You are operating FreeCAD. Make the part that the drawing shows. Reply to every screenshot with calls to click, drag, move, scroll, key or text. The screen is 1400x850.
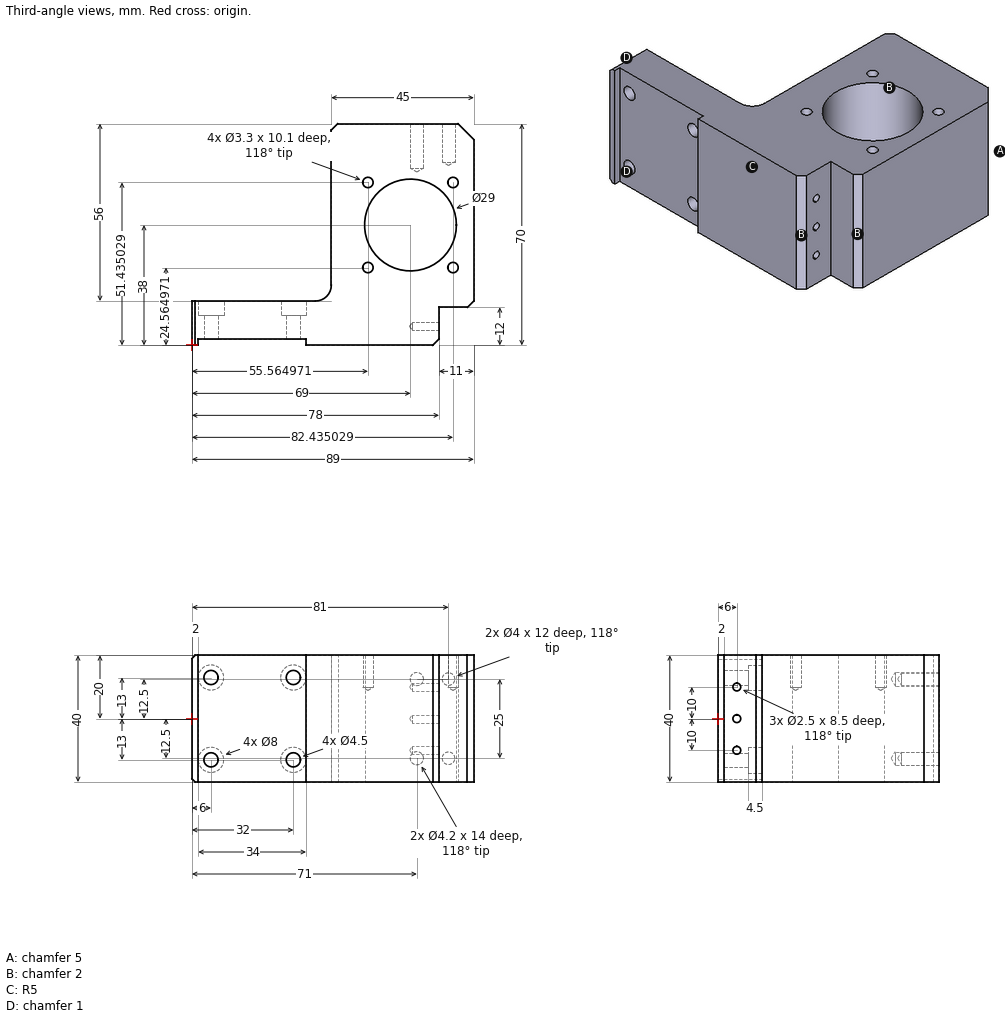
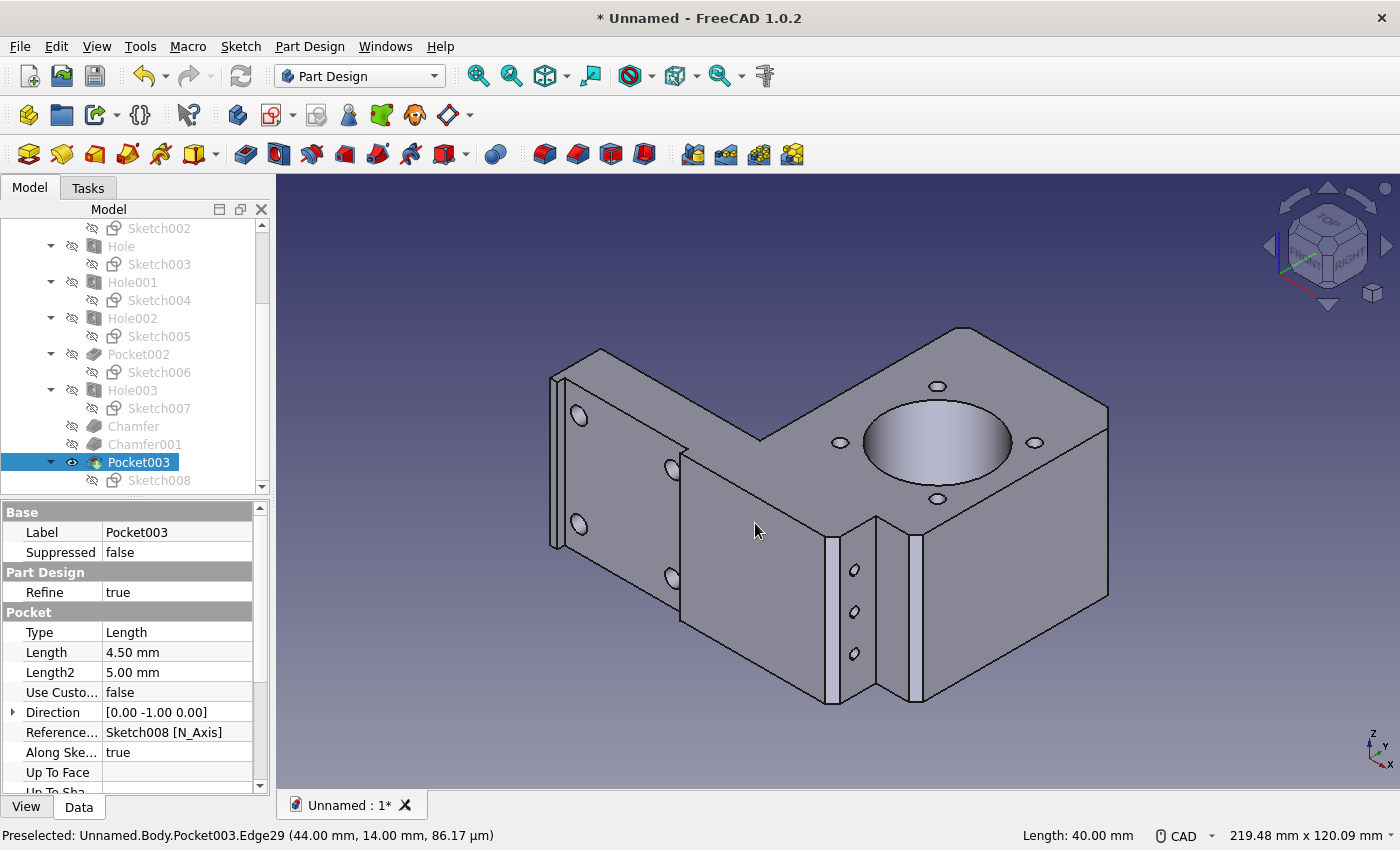
click(545, 154)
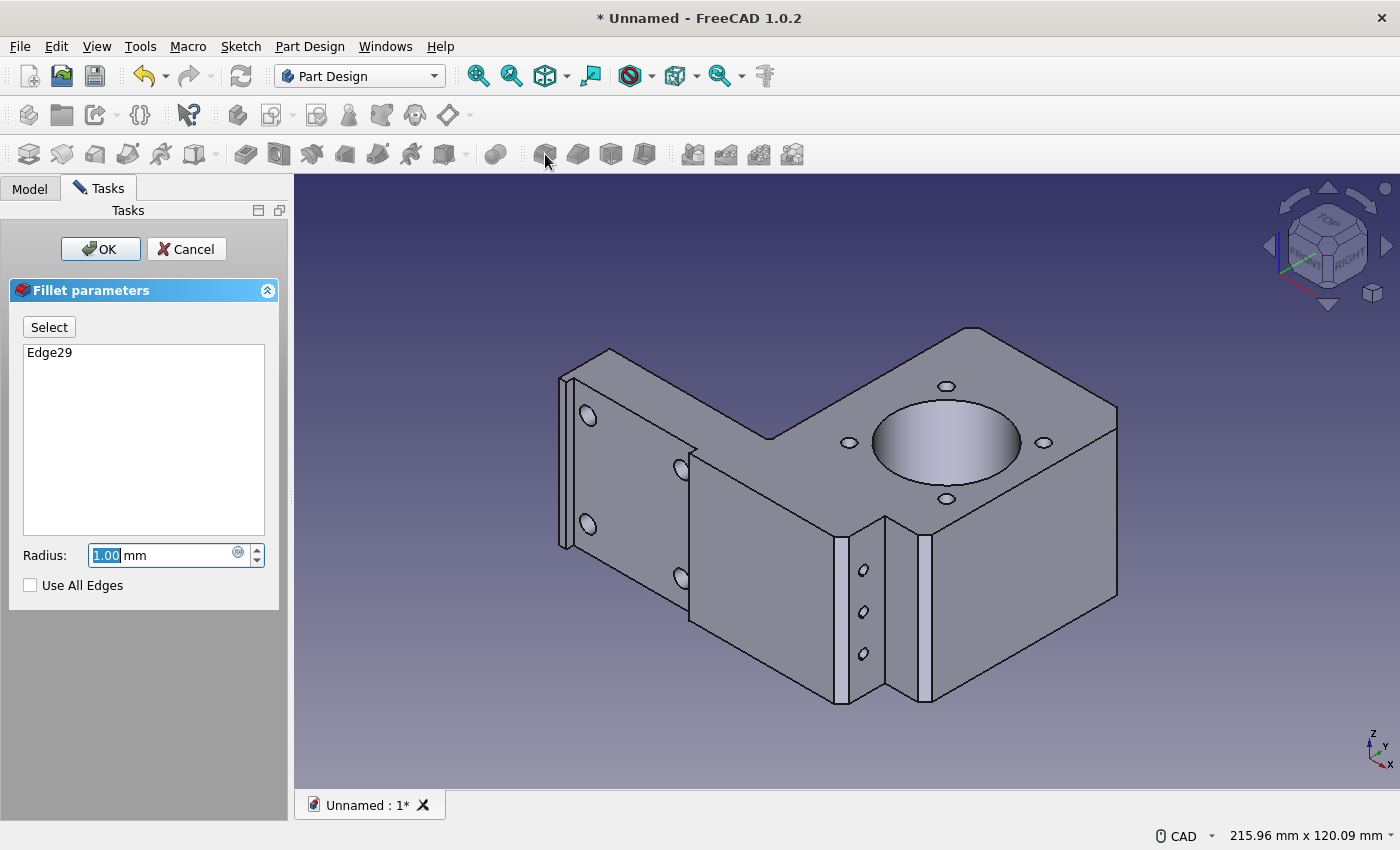
text(5)
key(Tab)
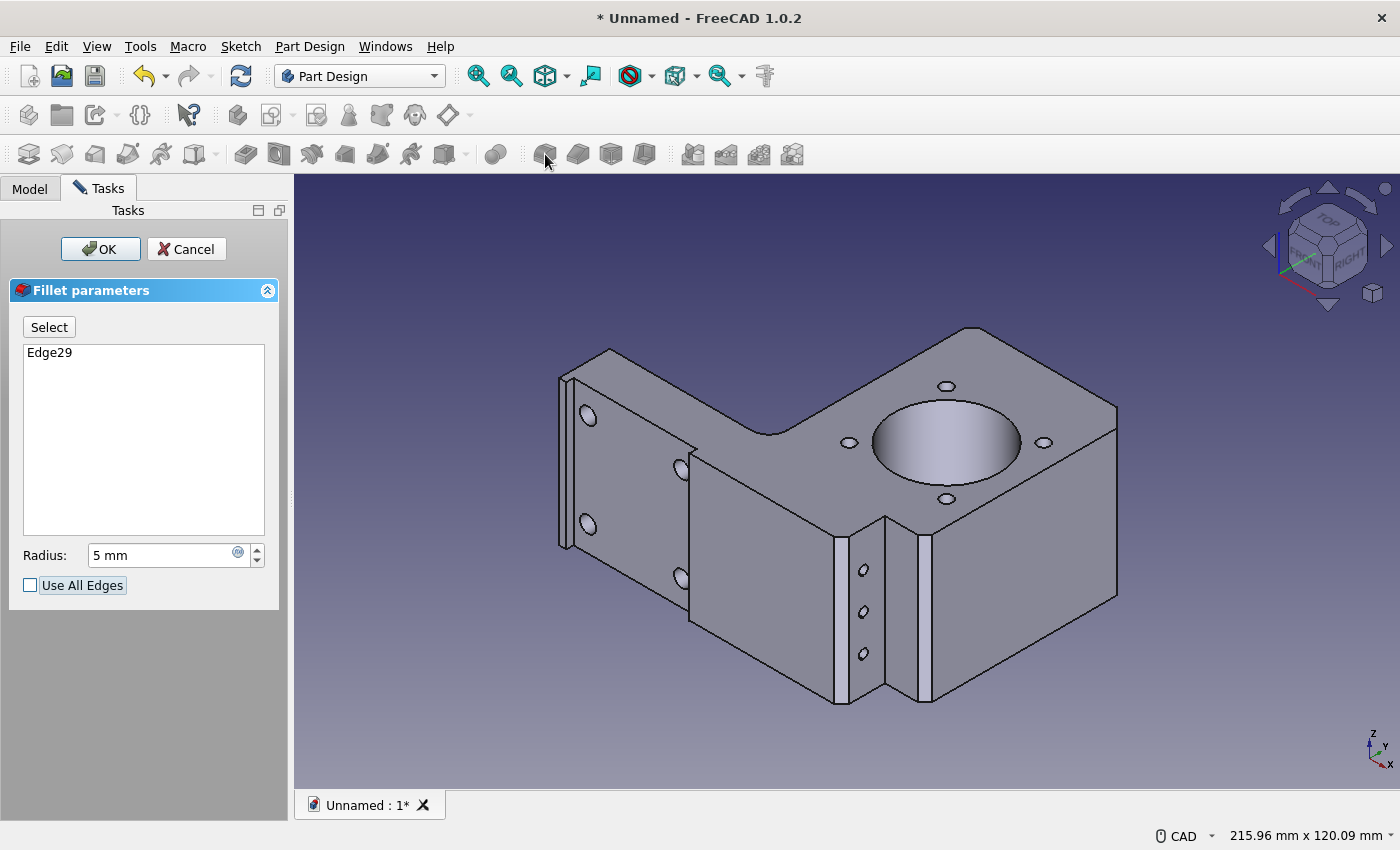
click(101, 249)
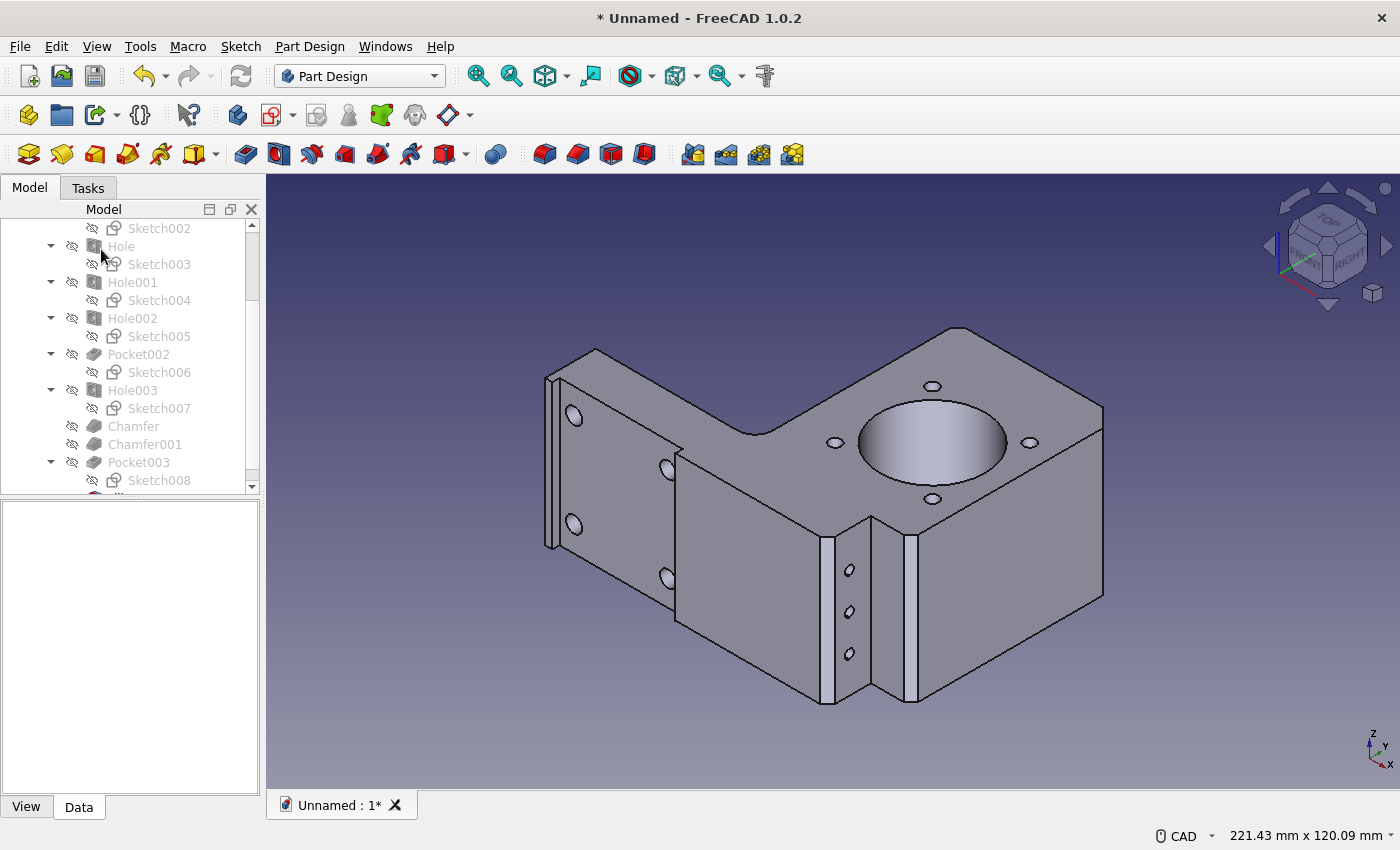
key(2)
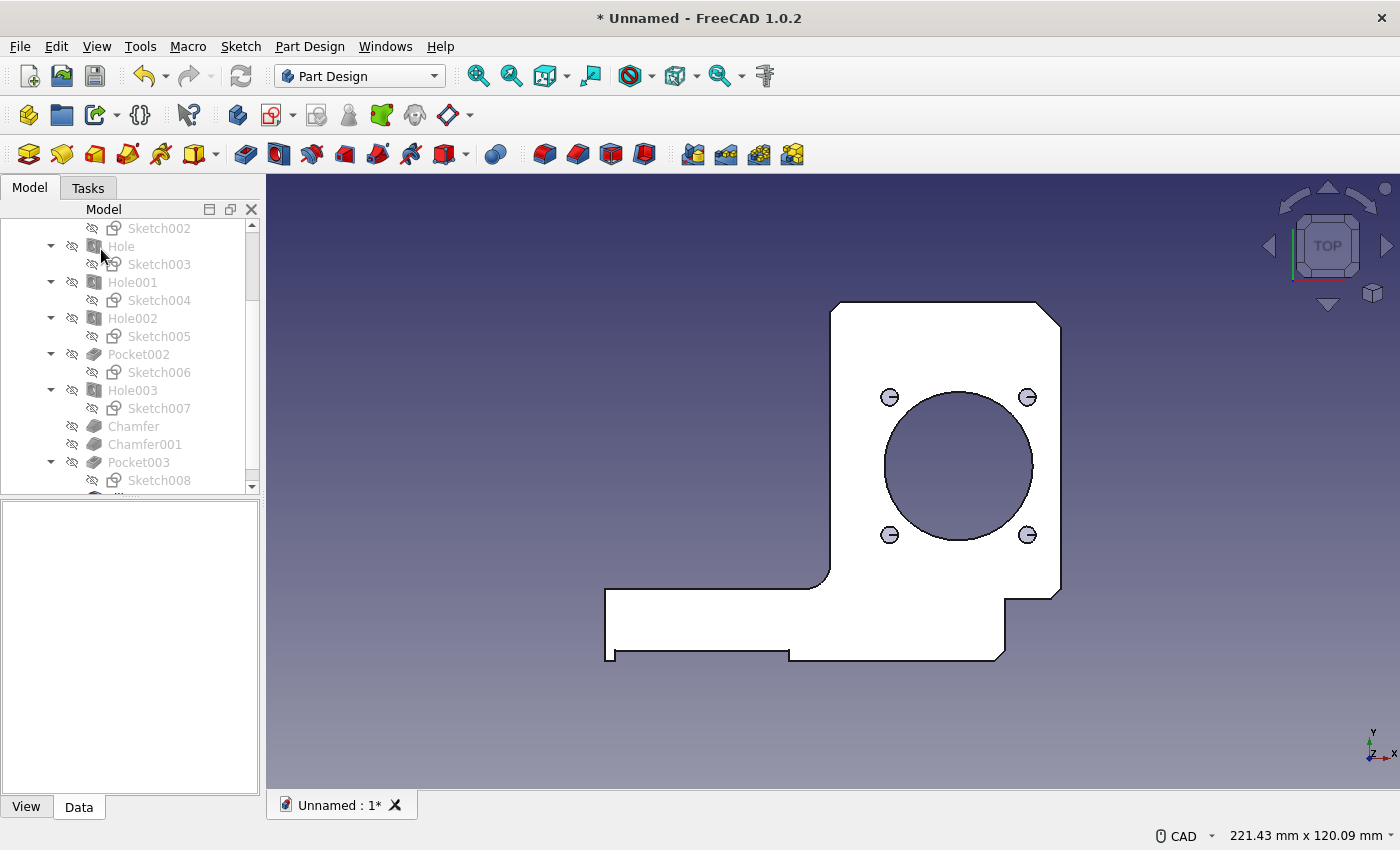
click(605, 624)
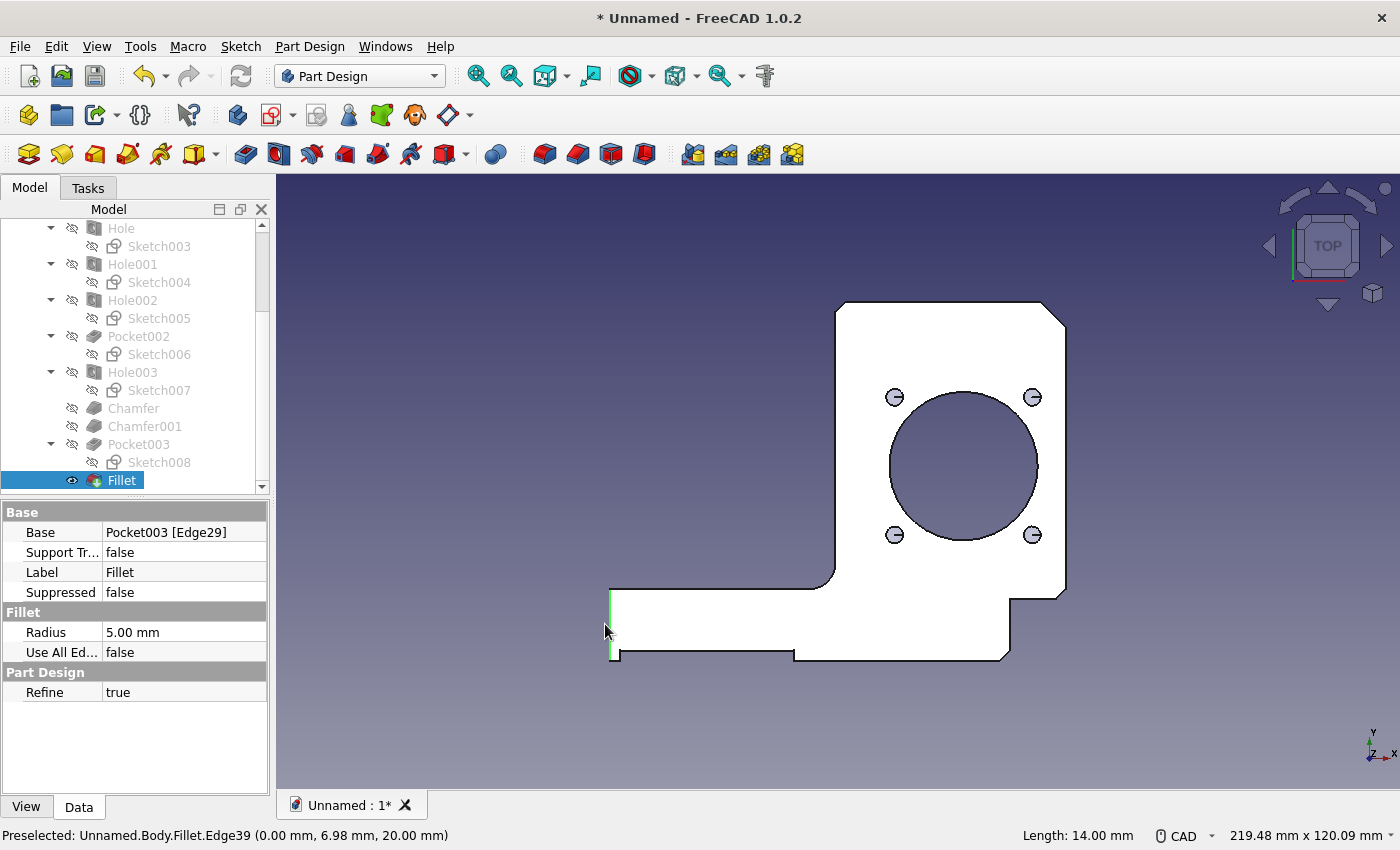
key(0)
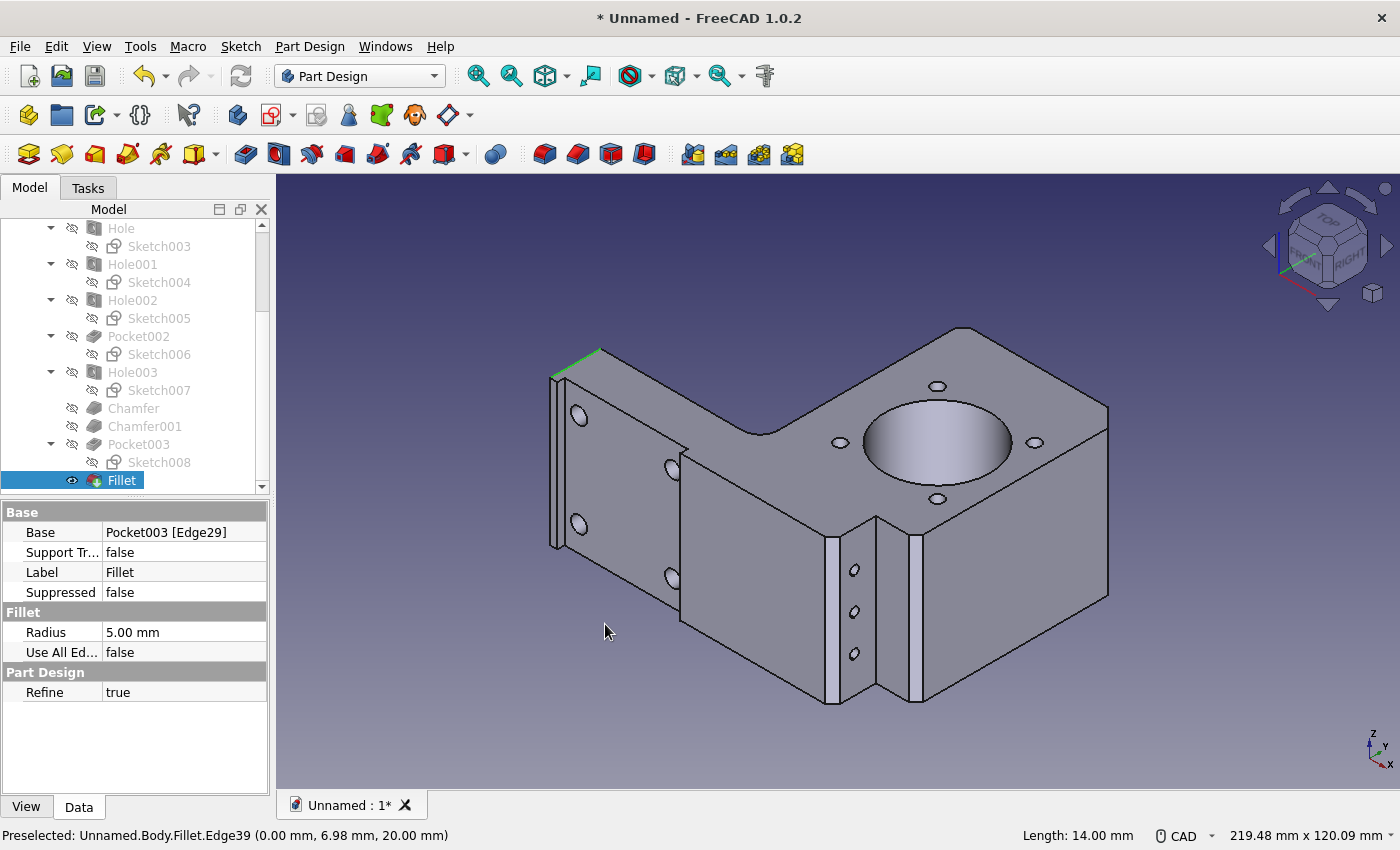
key(1)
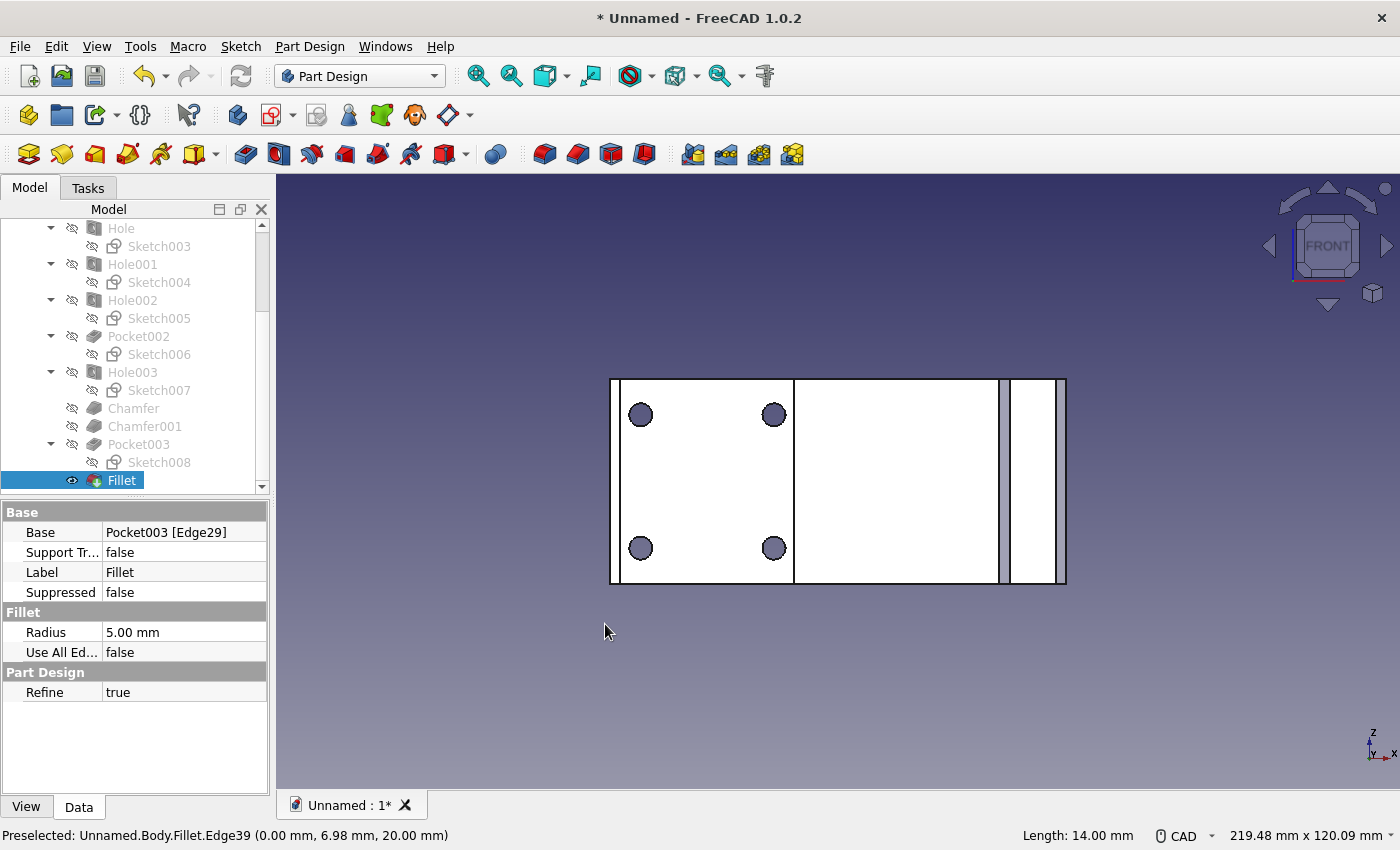
click(479, 76)